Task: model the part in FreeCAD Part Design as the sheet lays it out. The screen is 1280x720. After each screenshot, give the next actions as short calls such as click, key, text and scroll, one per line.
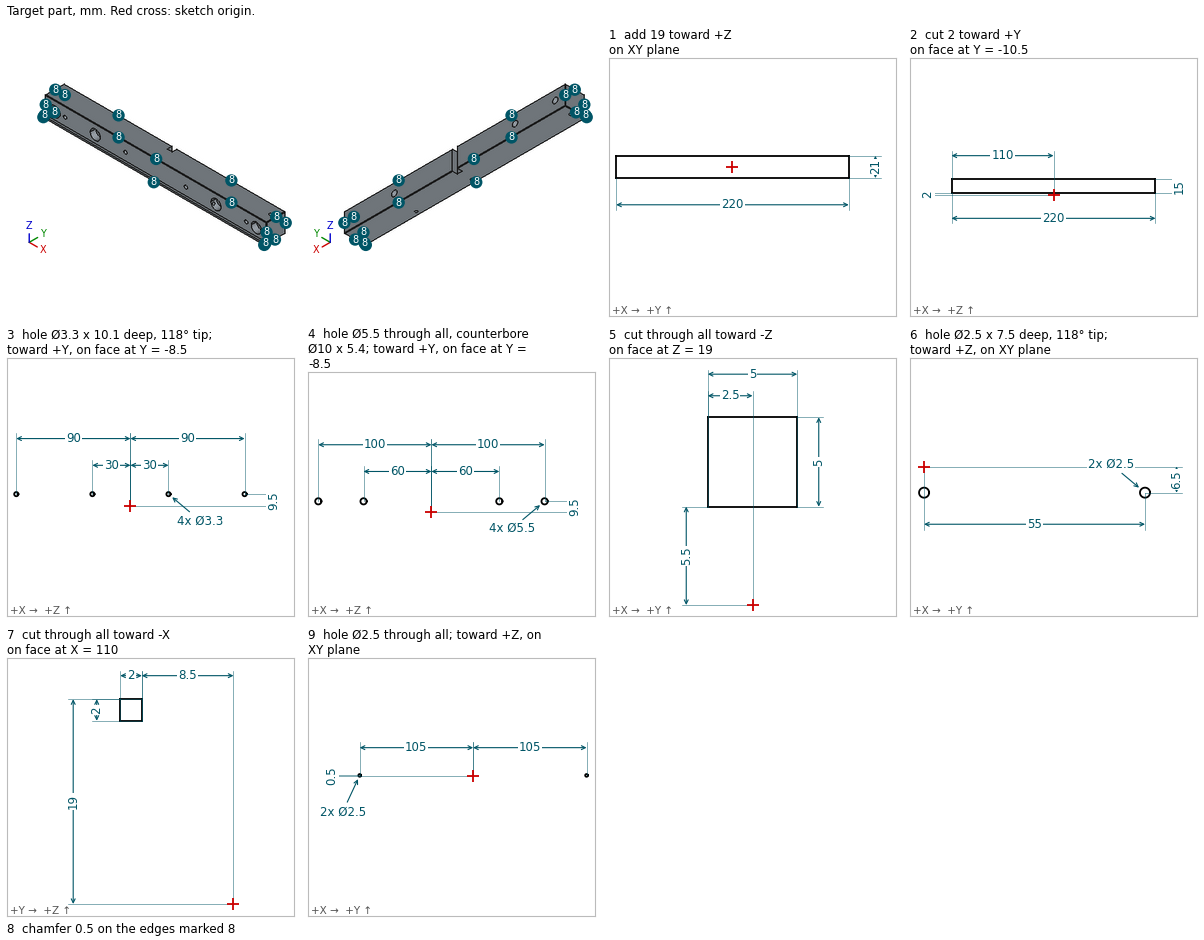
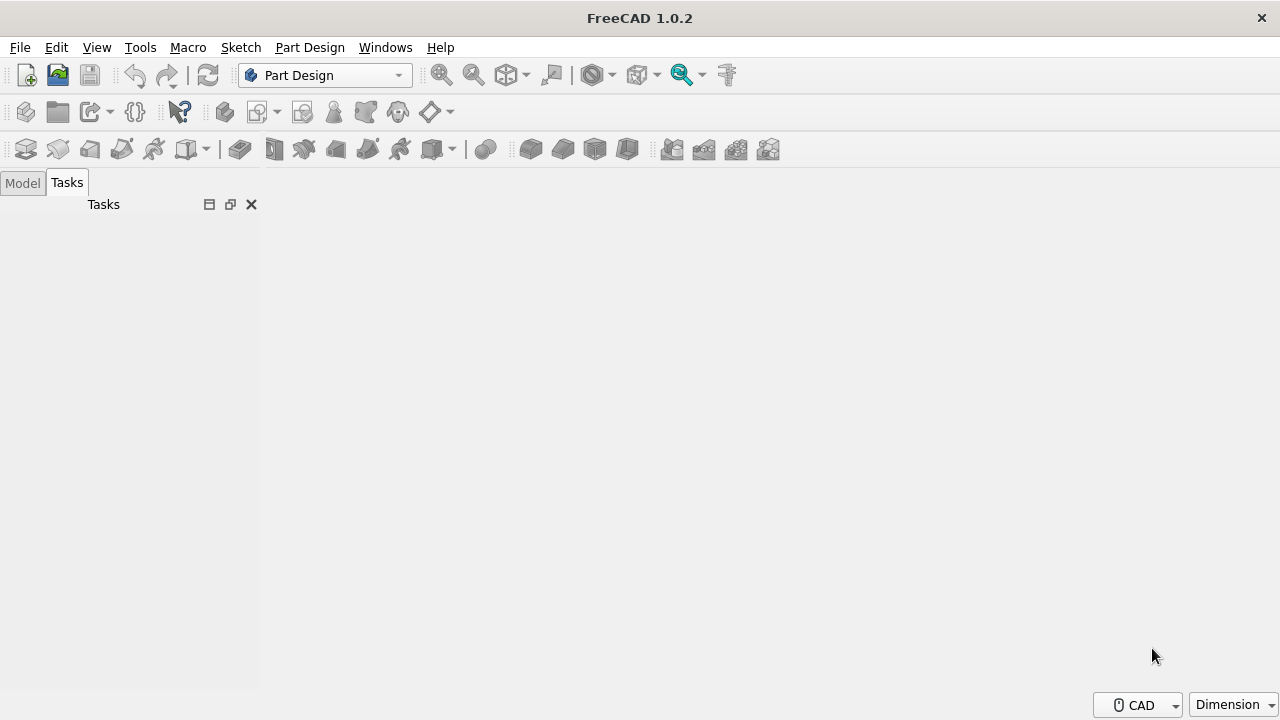
click(26, 76)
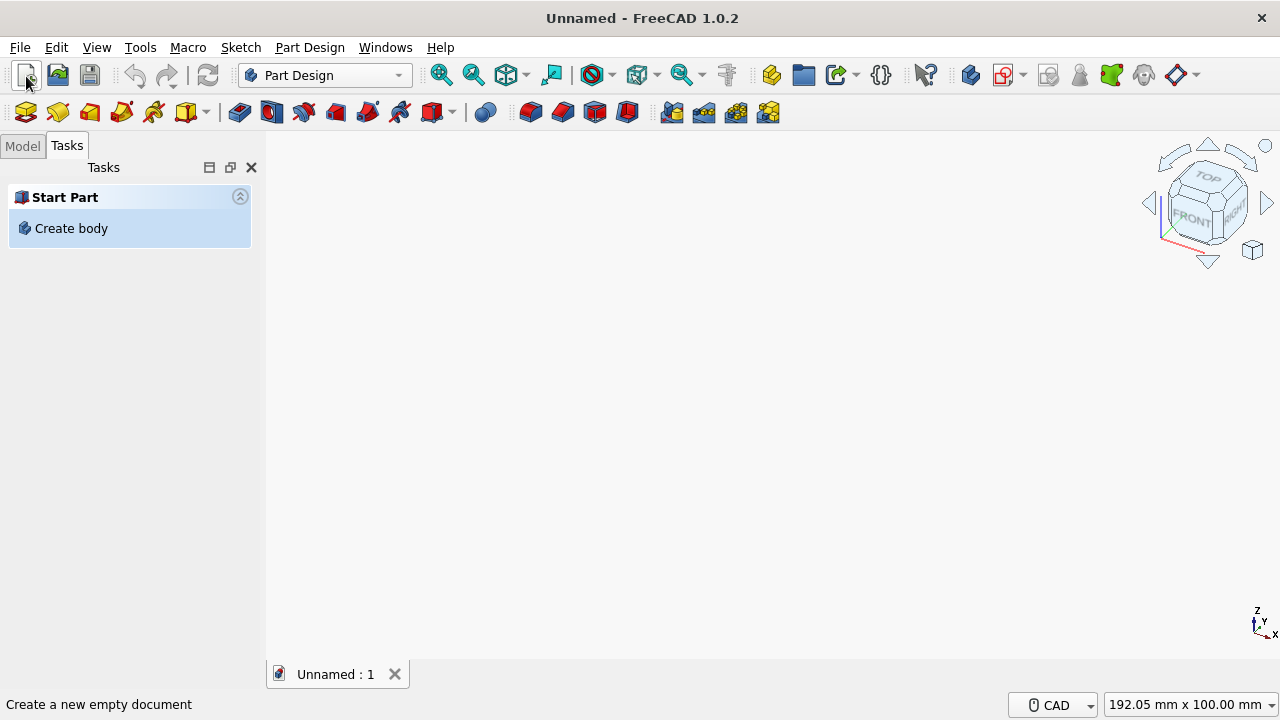
click(1004, 76)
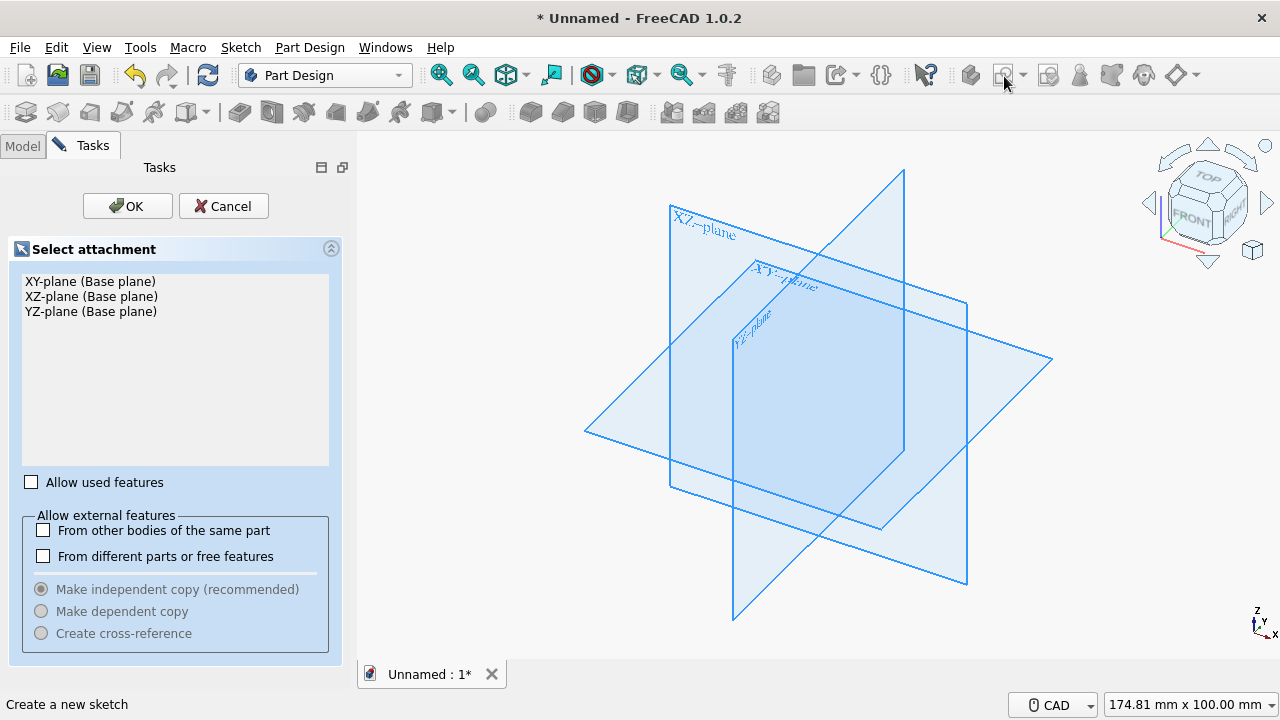
click(82, 282)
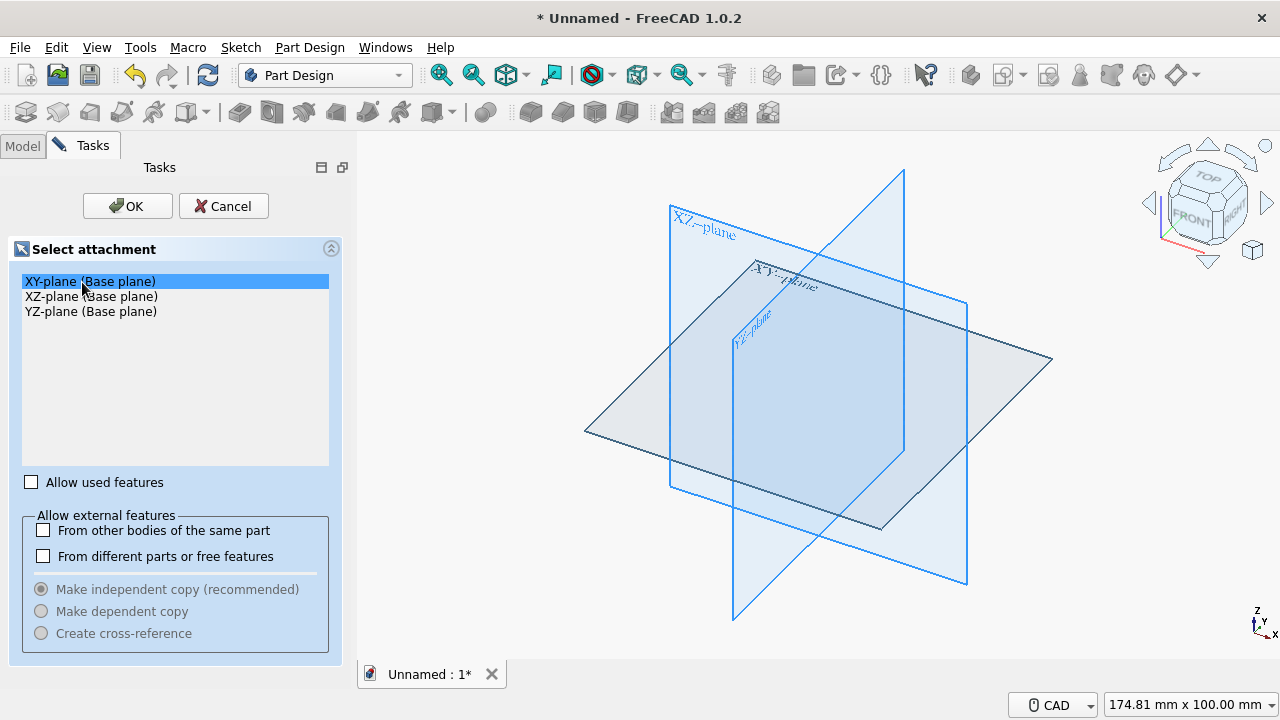
click(128, 206)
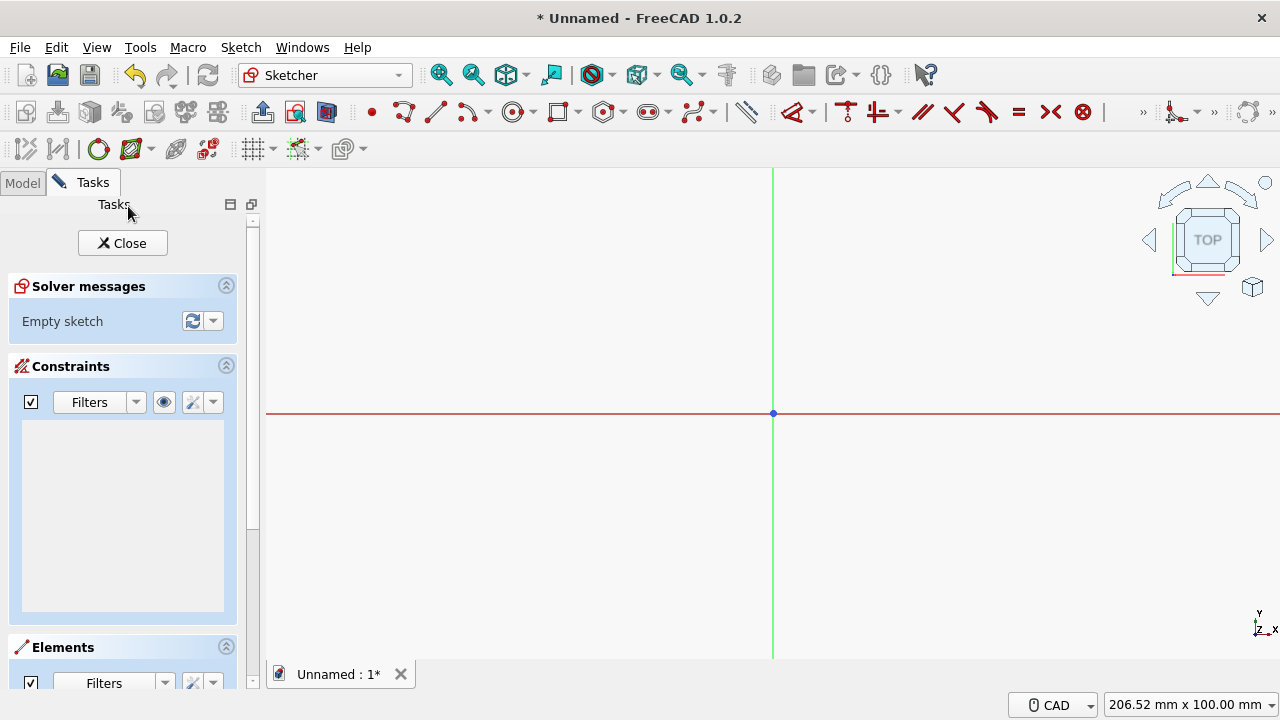
scroll(621, 414, down, 3)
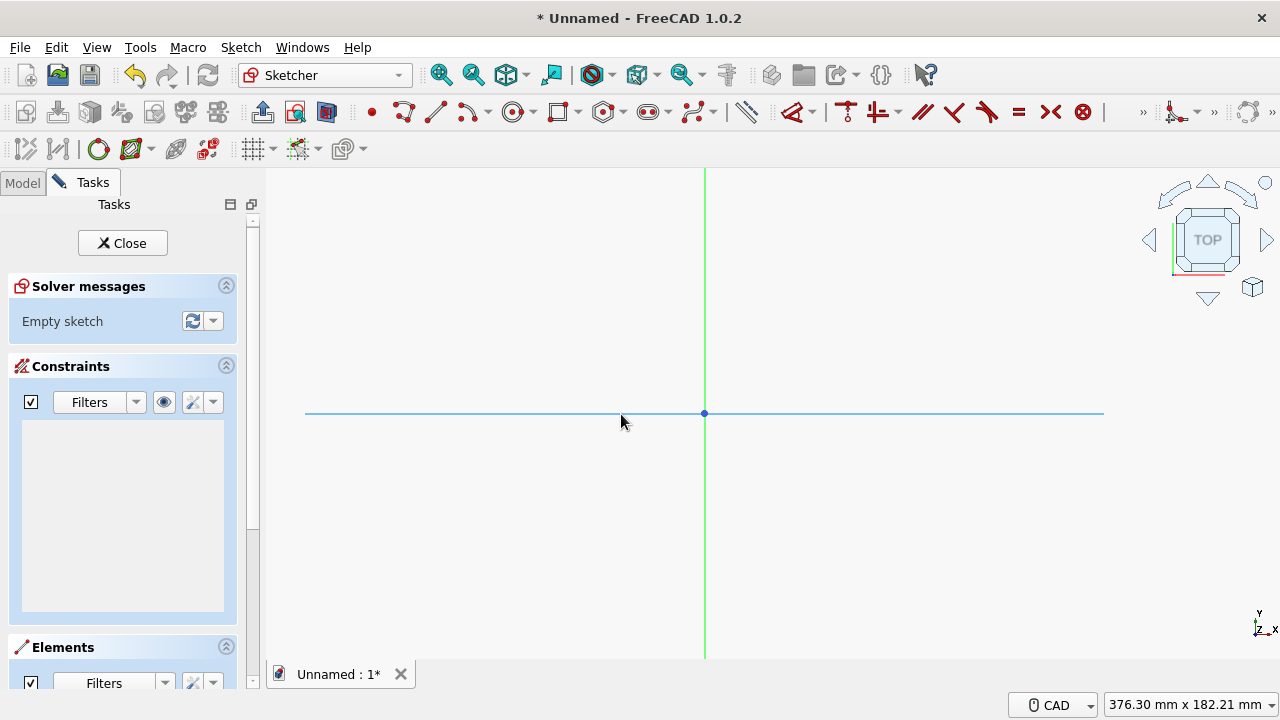
click(580, 112)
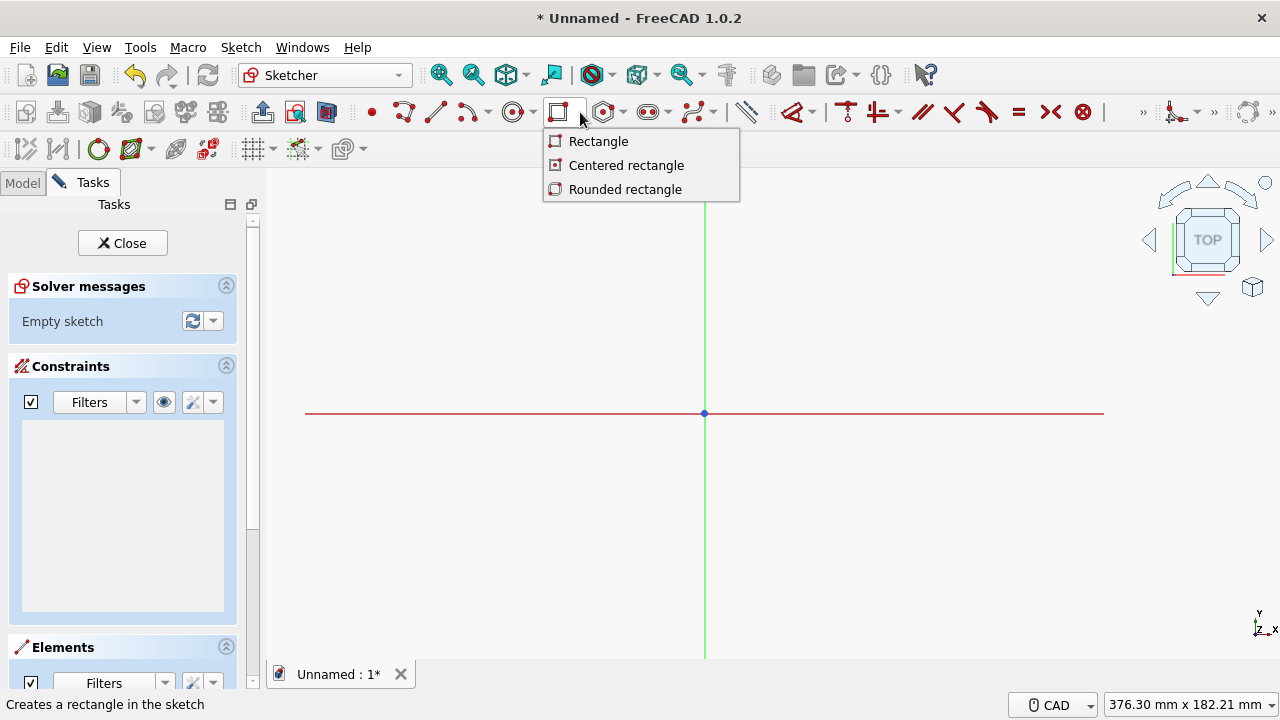
click(642, 165)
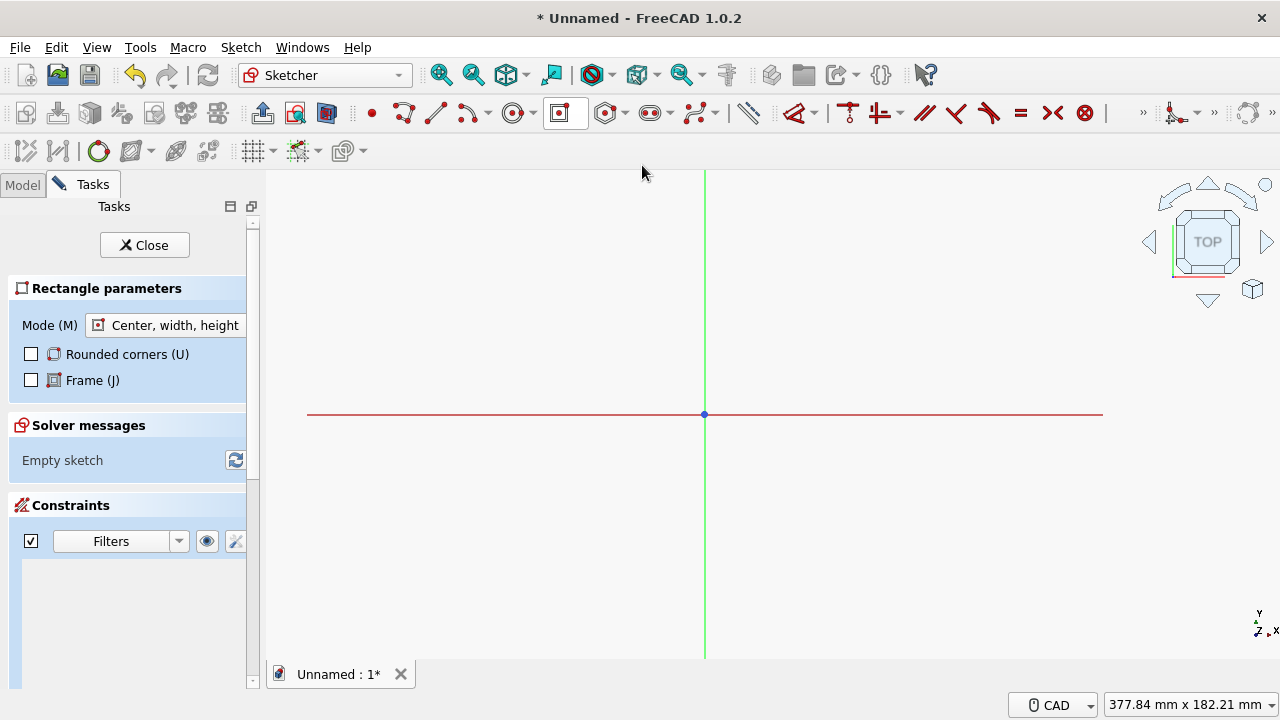
click(705, 415)
move(1000, 387)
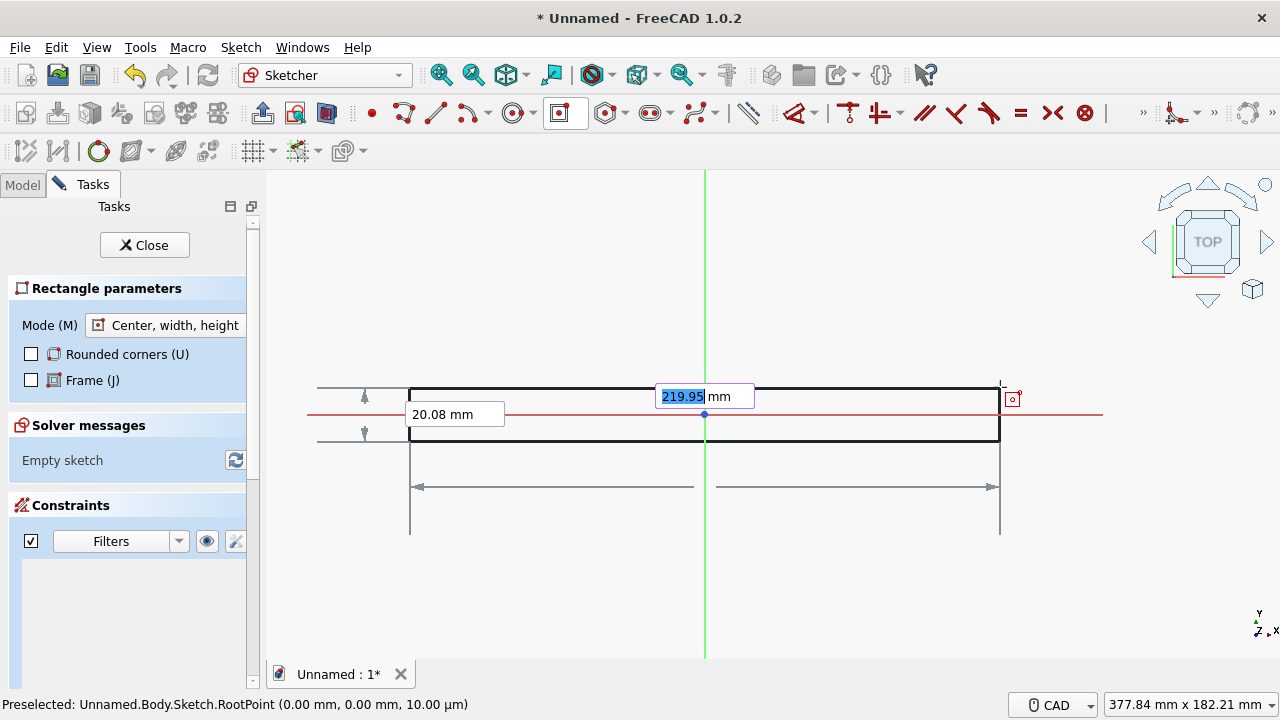
text(220)
key(Tab)
text(21)
key(Return)
key(Escape)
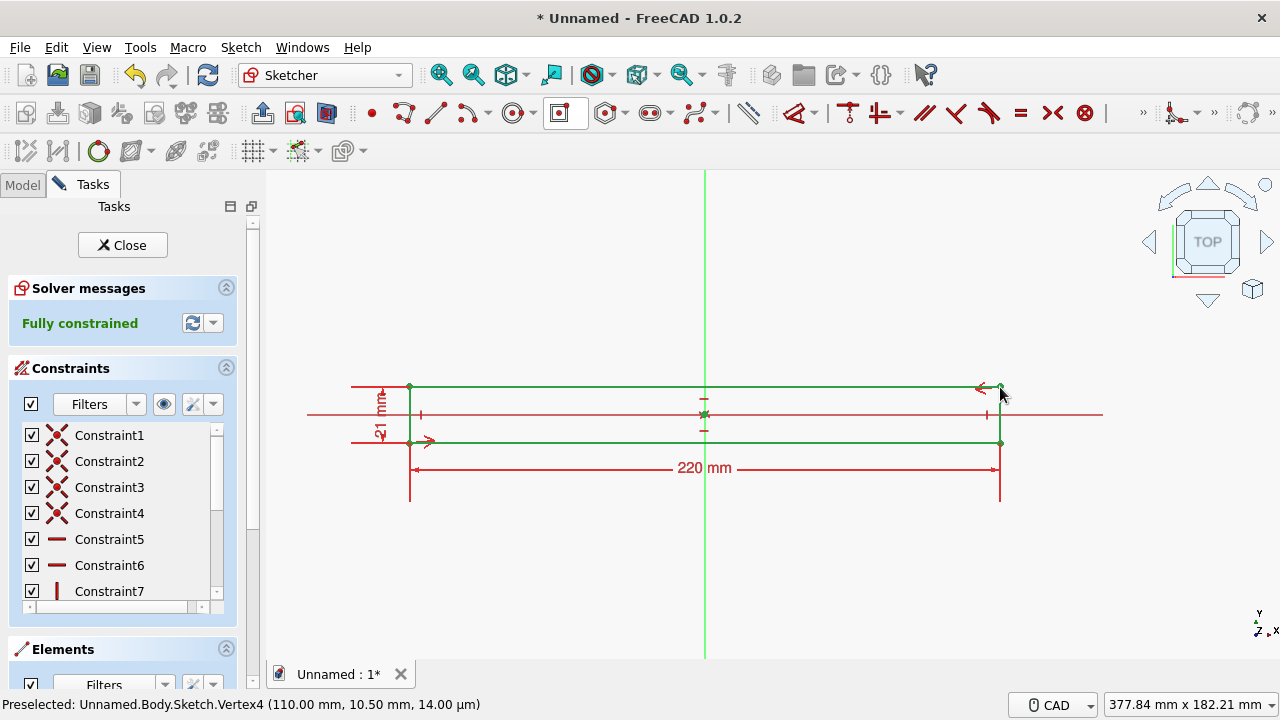
click(123, 245)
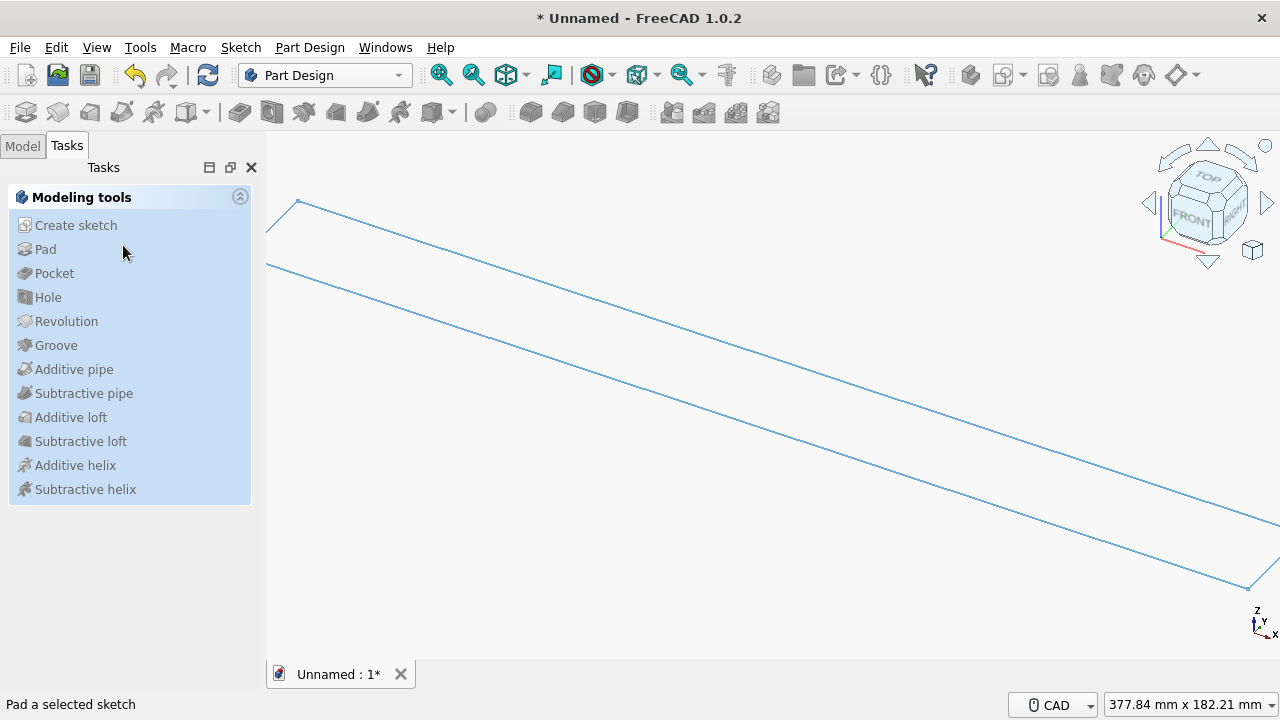
click(26, 112)